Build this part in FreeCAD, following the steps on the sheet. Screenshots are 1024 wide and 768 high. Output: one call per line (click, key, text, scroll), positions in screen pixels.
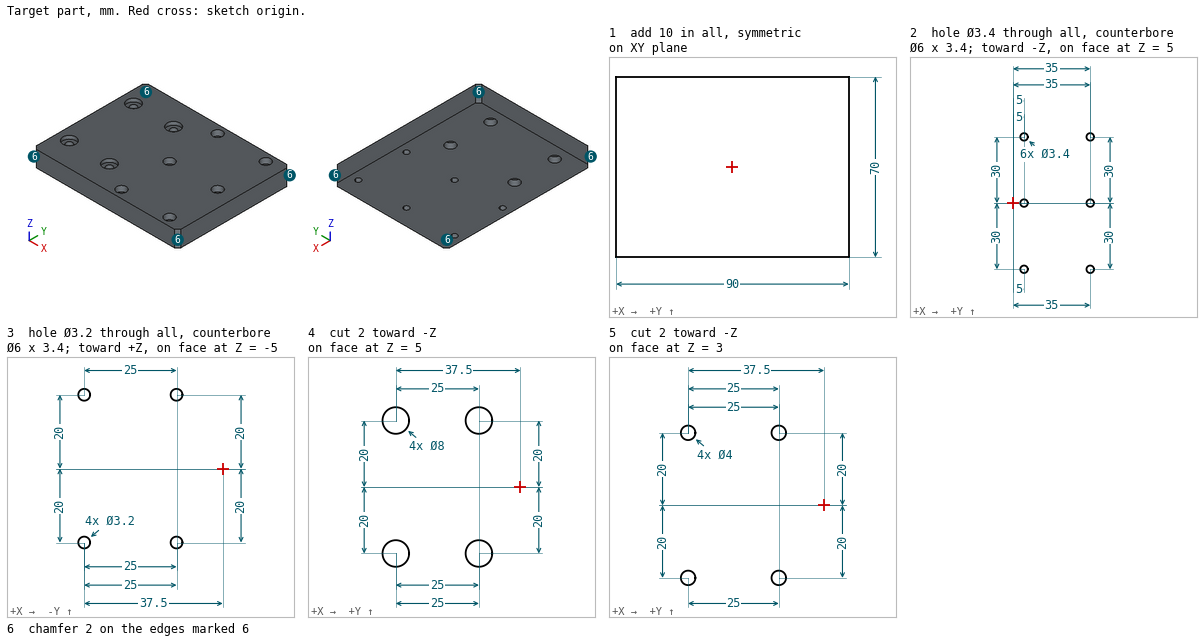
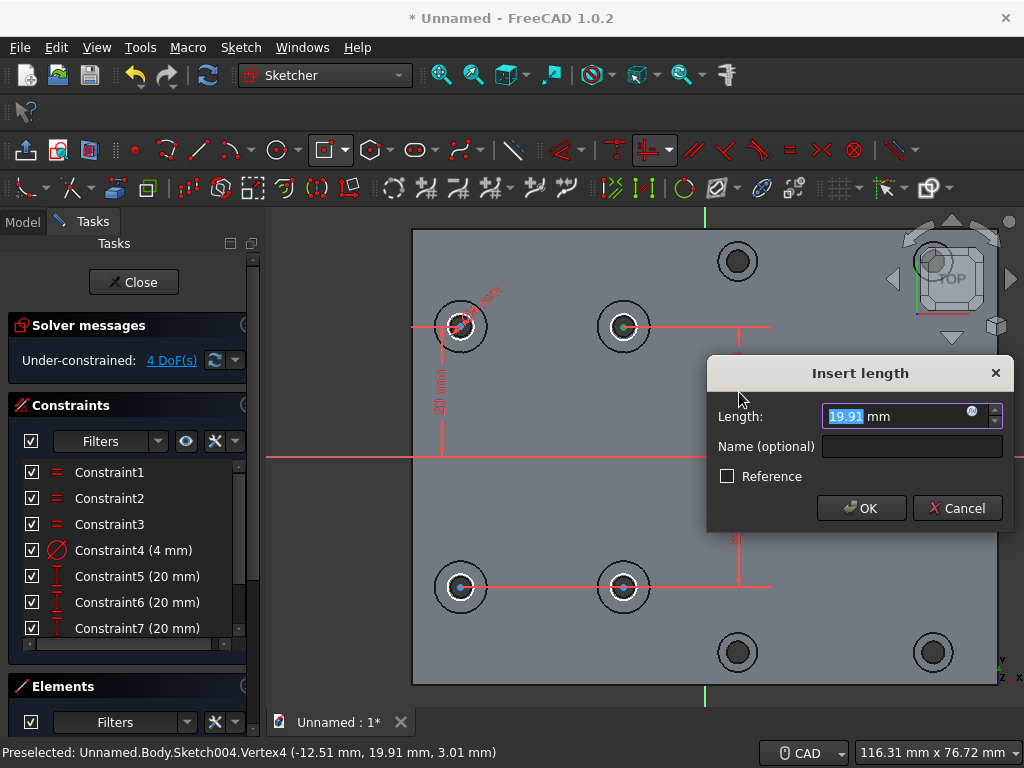
text(20)
key(Return)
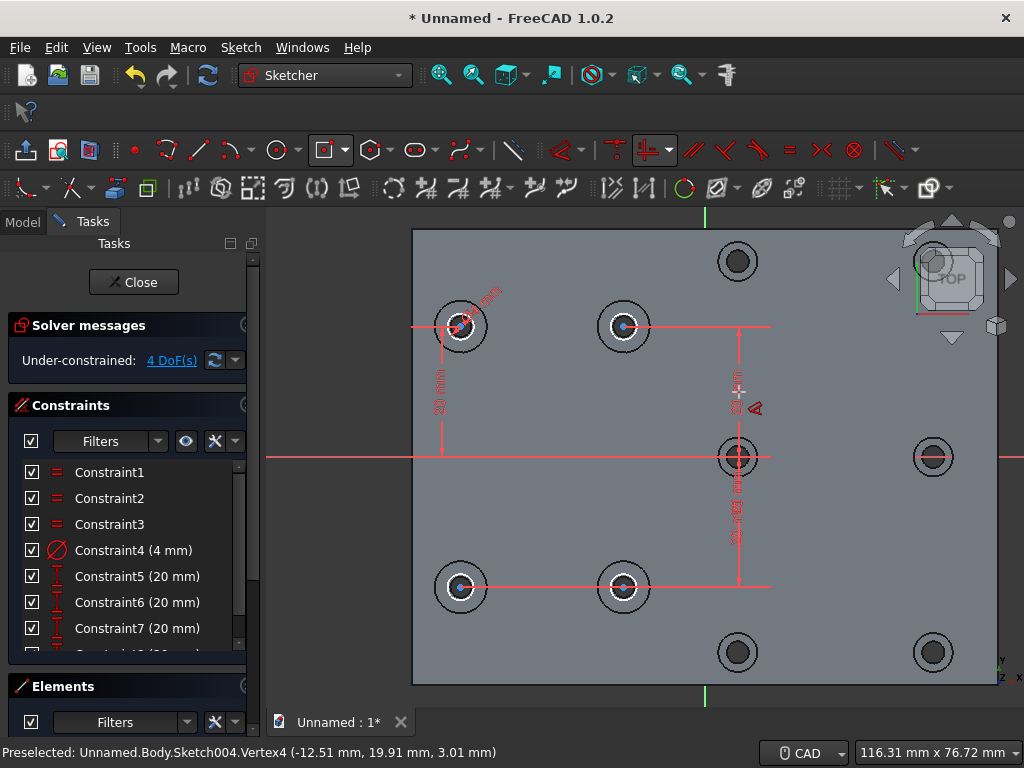
click(461, 587)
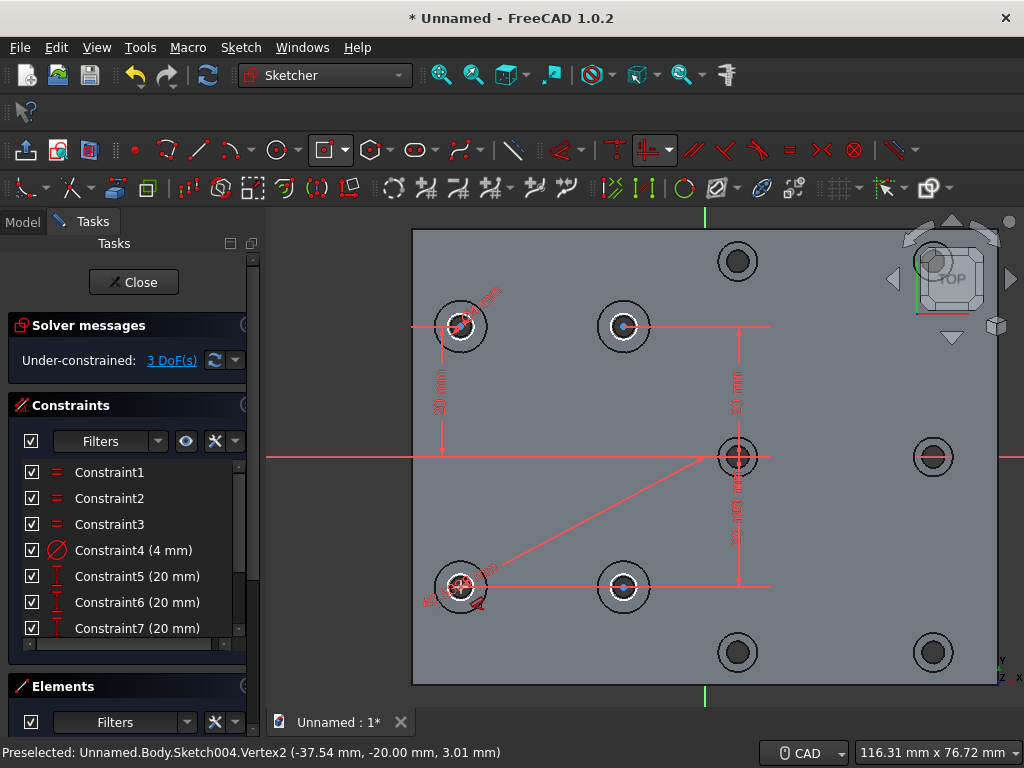
click(624, 587)
click(542, 621)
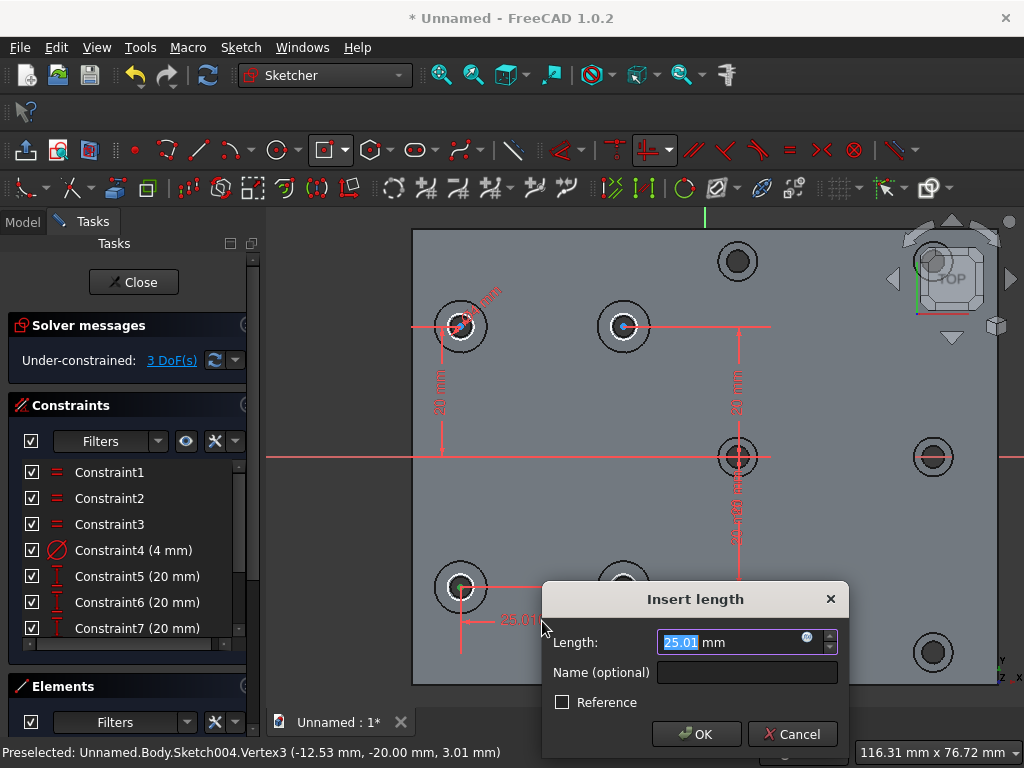
text(25)
key(Return)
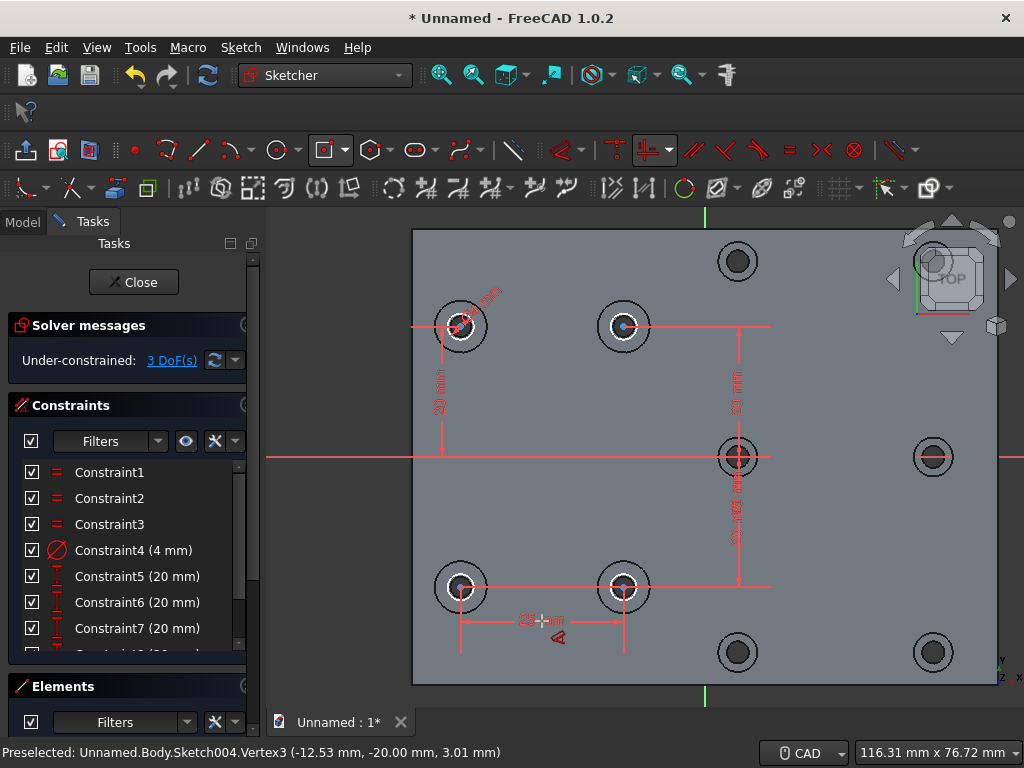
click(461, 327)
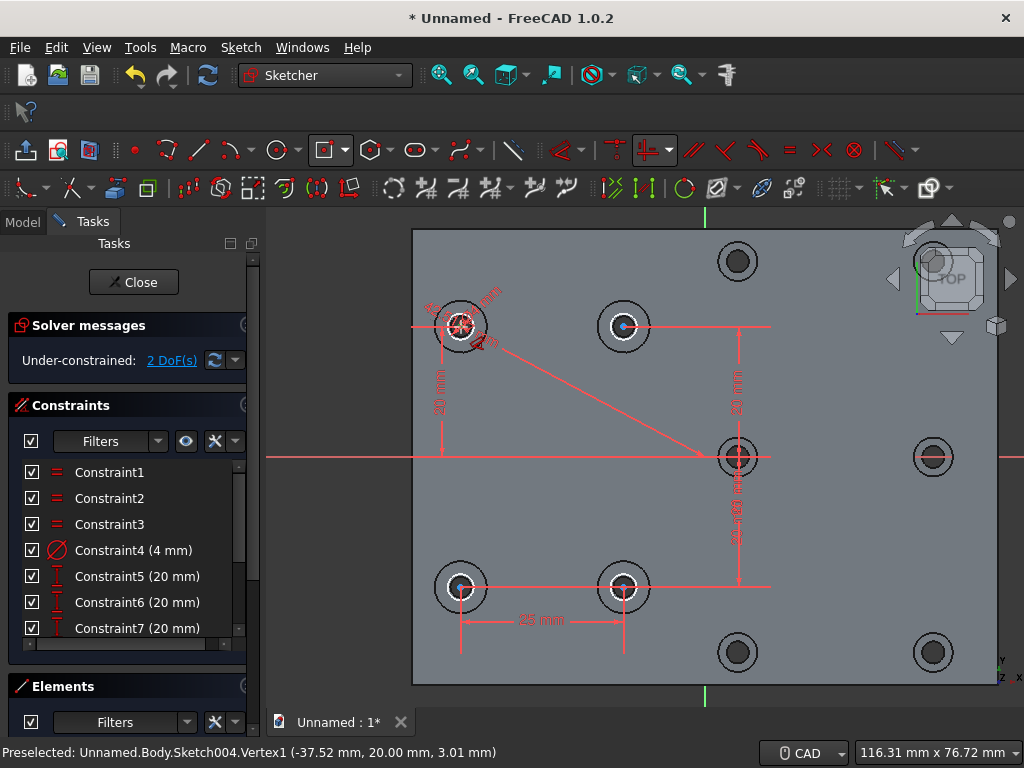
click(624, 587)
click(580, 293)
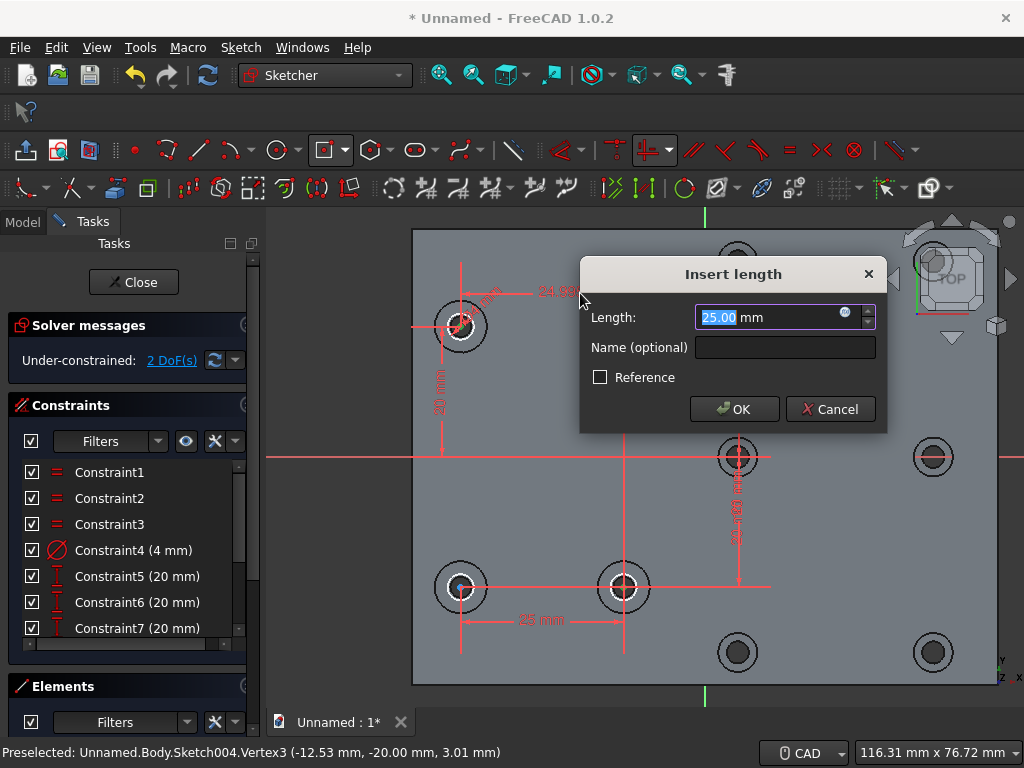
text(25)
key(Return)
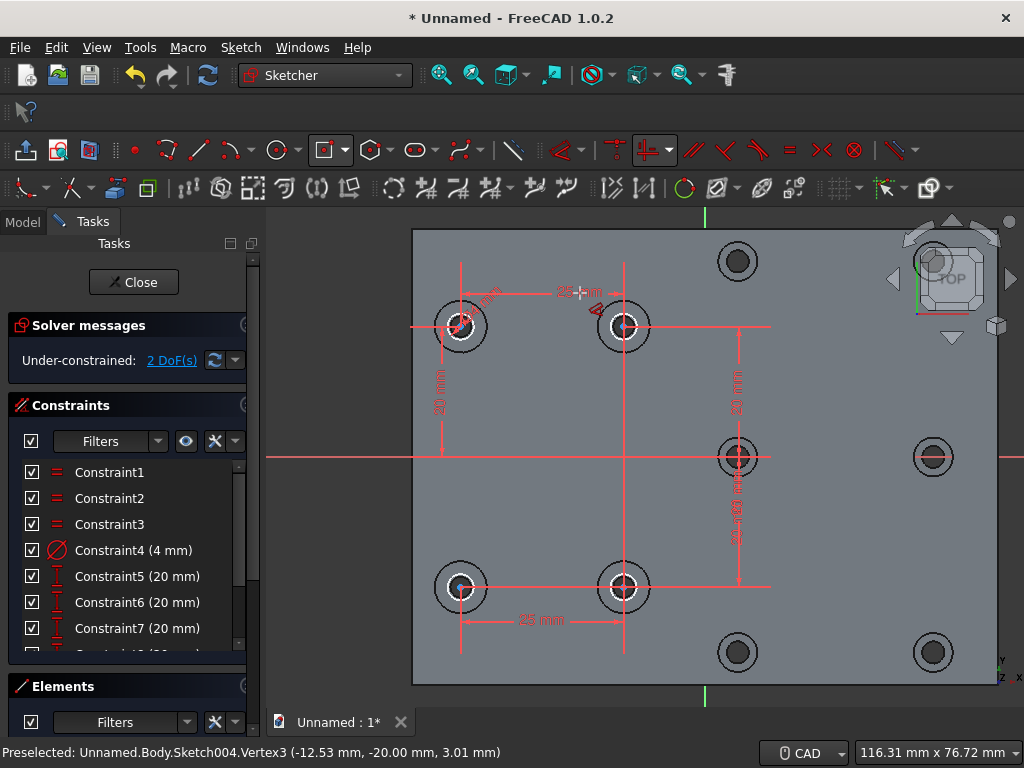
click(461, 327)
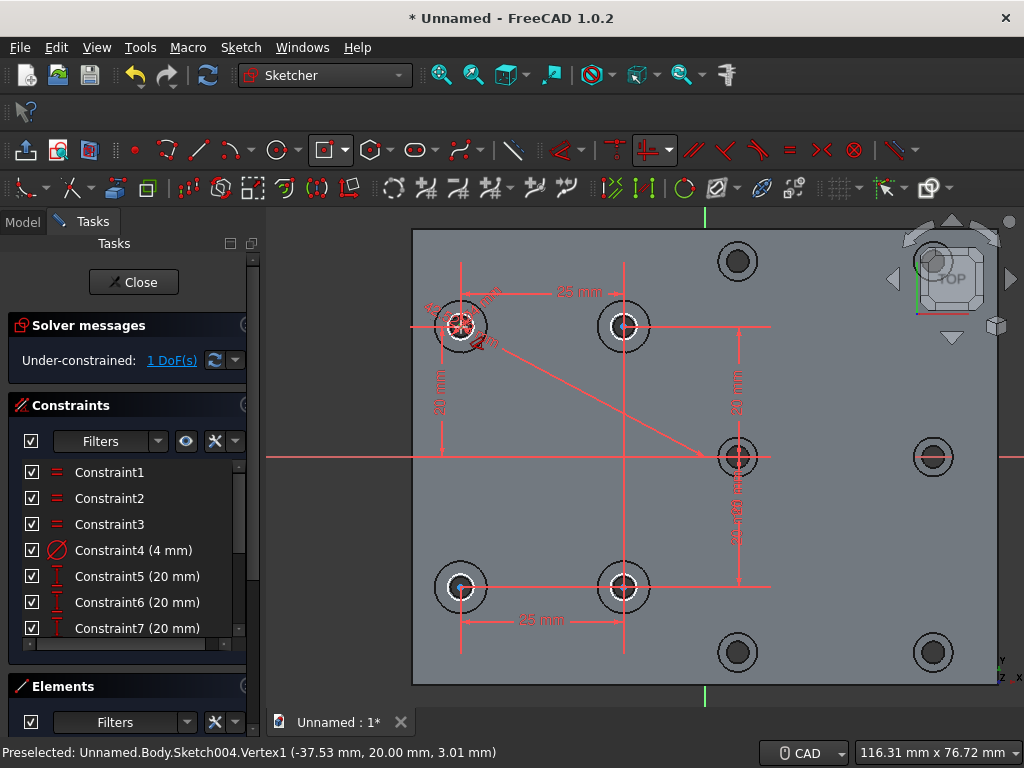
click(624, 327)
click(542, 361)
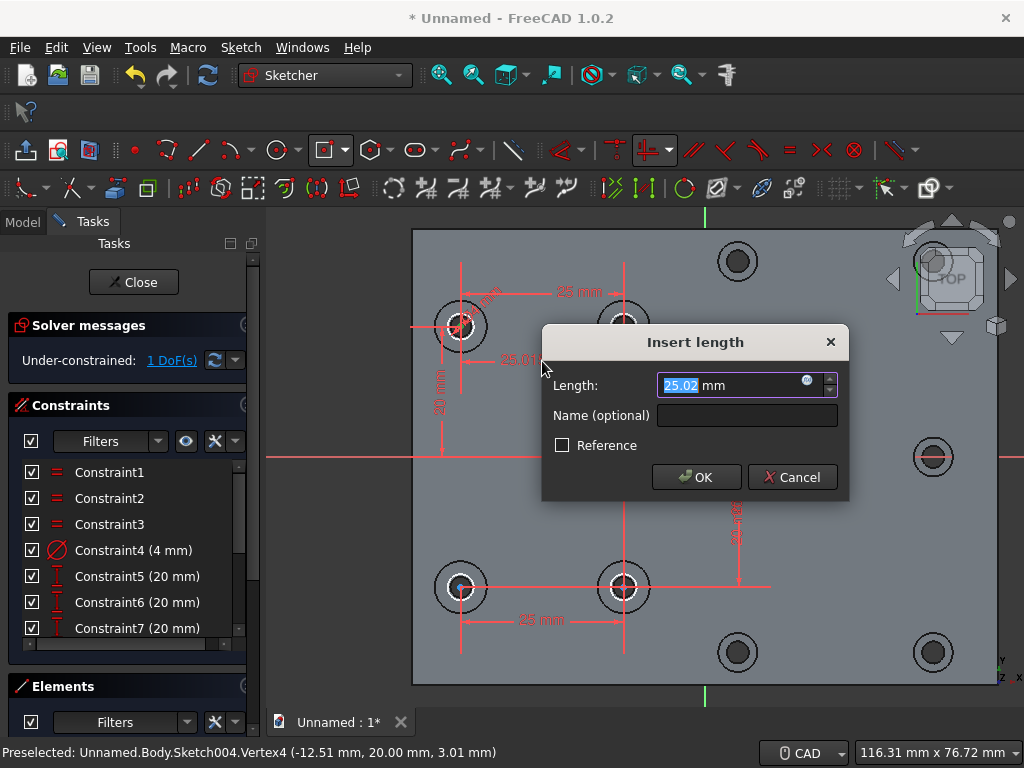
text(25)
key(Return)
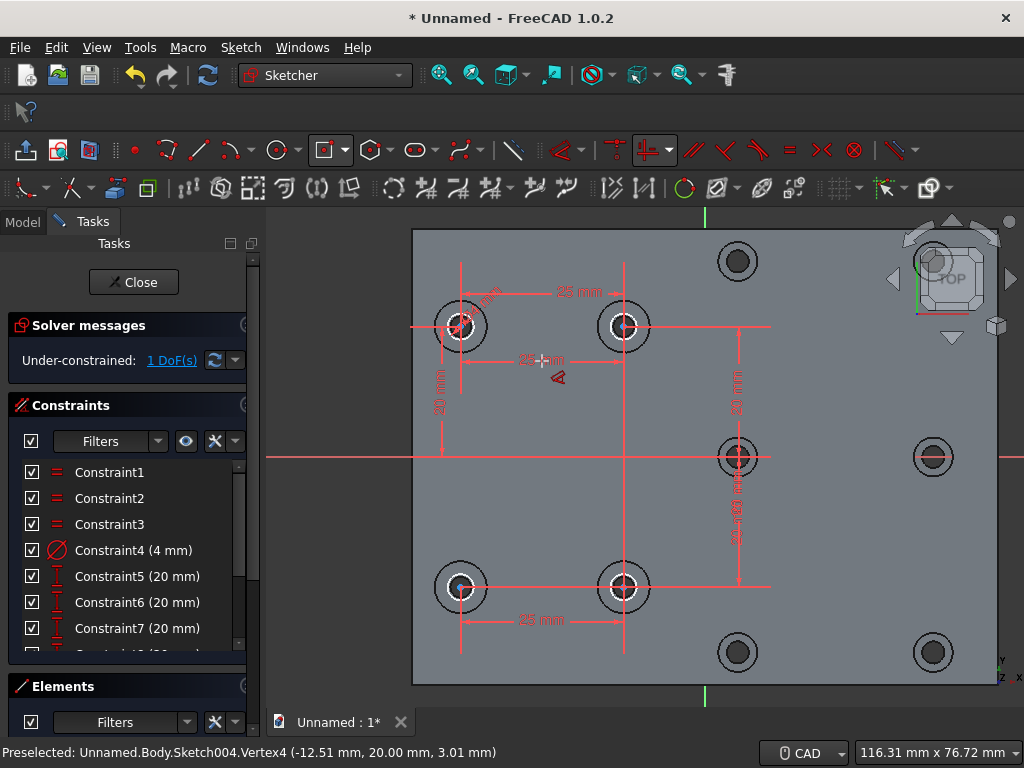
click(461, 327)
click(669, 293)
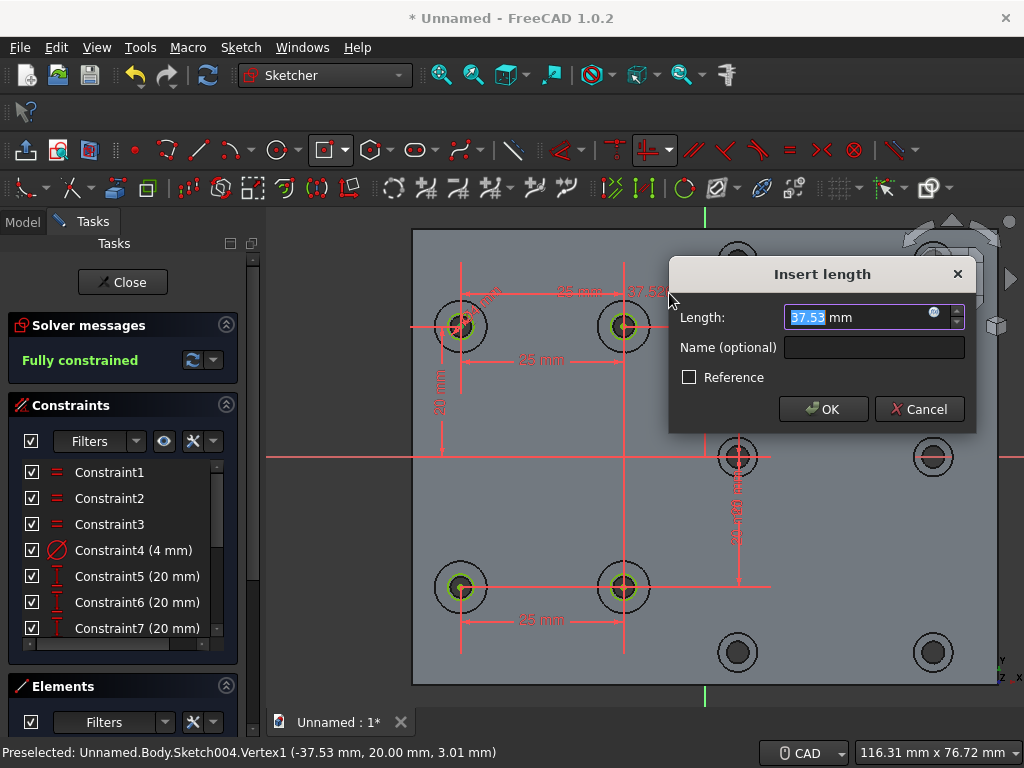
text(37.5)
key(Return)
key(Escape)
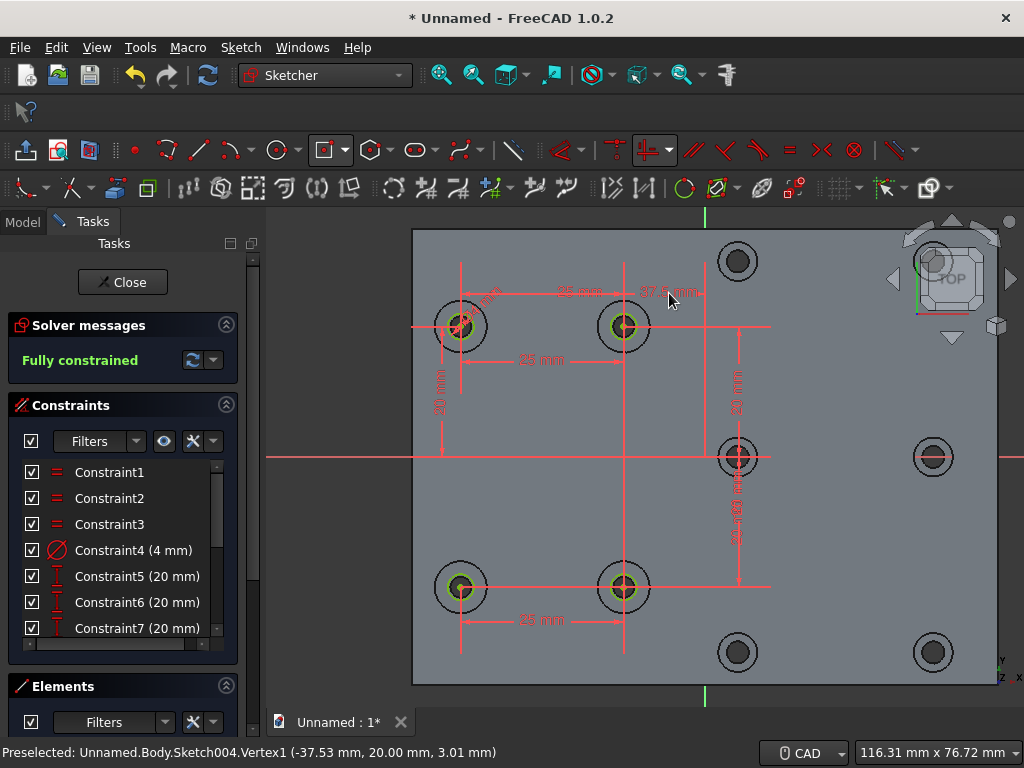
click(123, 282)